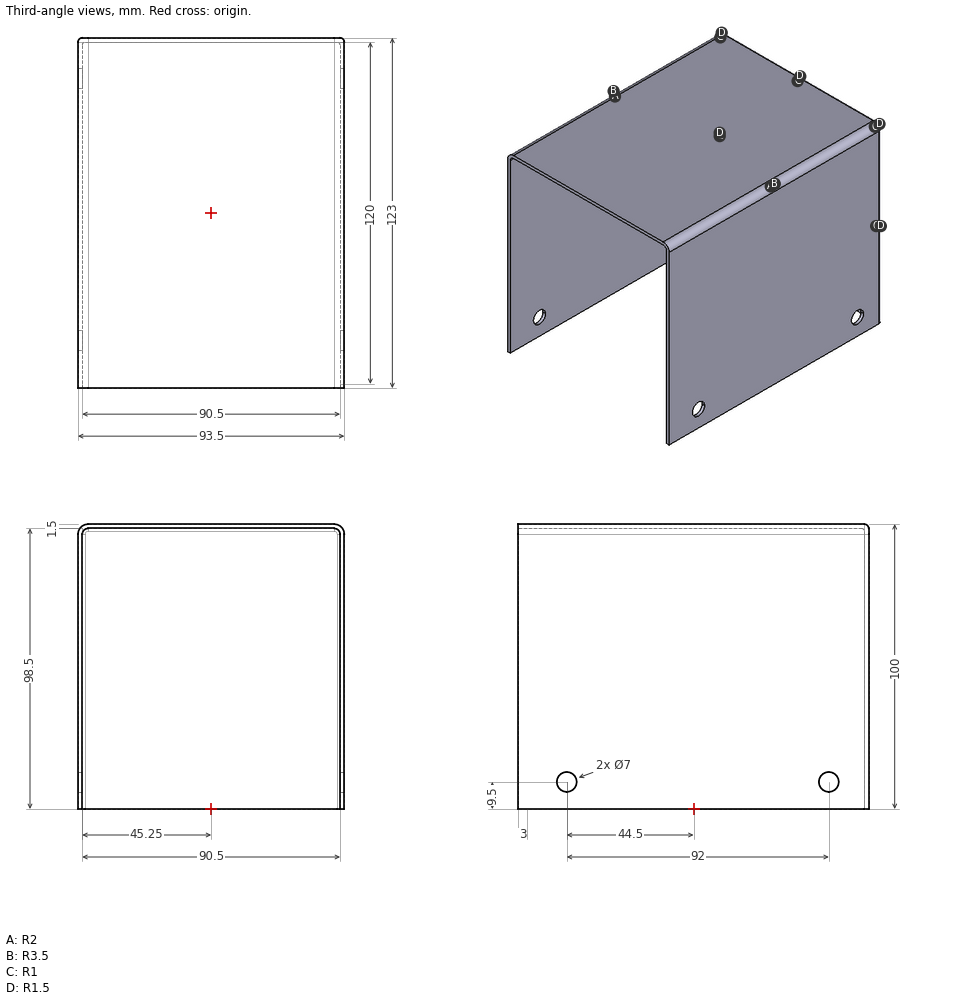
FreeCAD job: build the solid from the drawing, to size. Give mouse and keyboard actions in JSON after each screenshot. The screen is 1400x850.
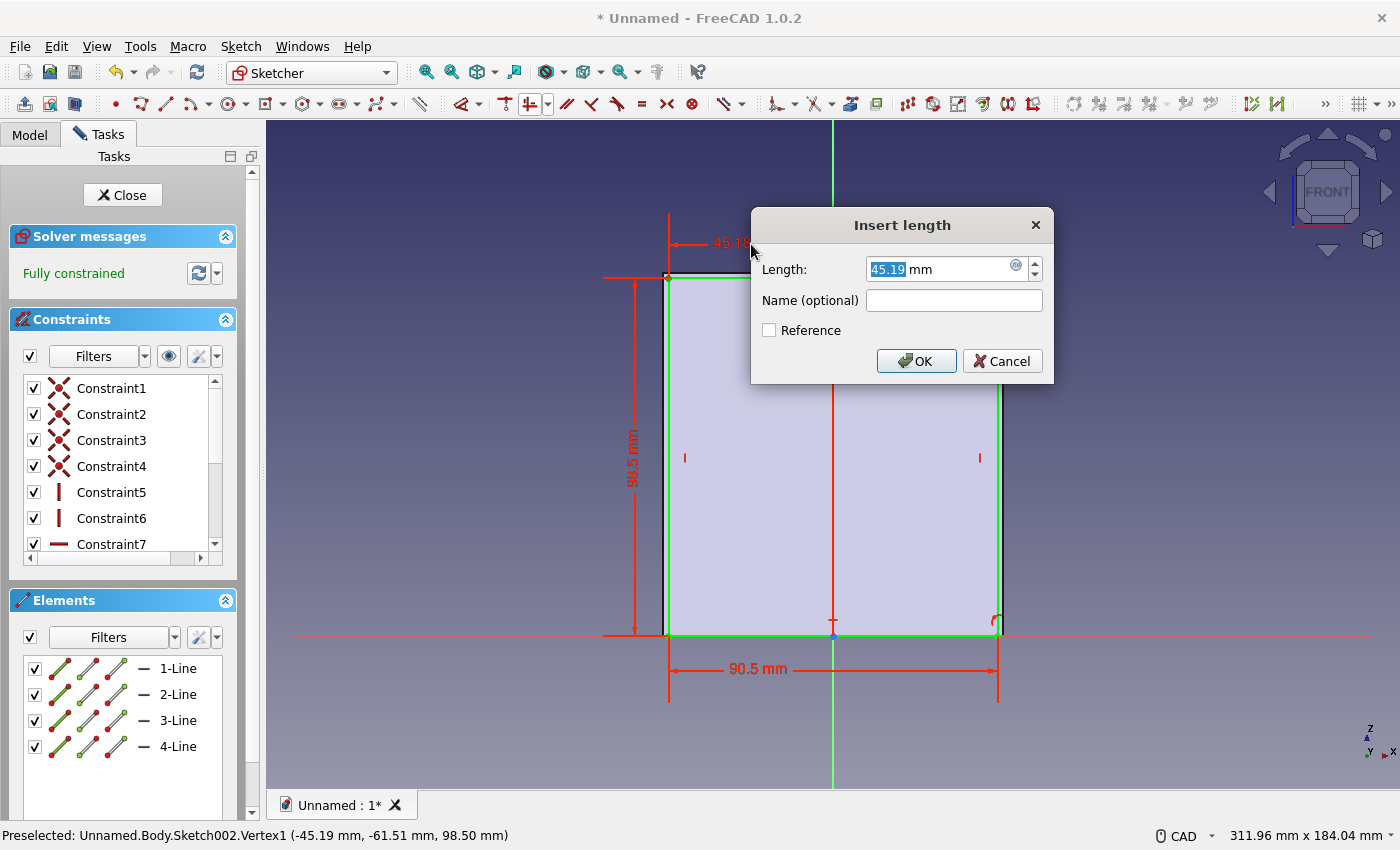
{"action": "type", "text": "45.25"}
{"action": "key", "text": "Return"}
{"action": "key", "text": "Escape"}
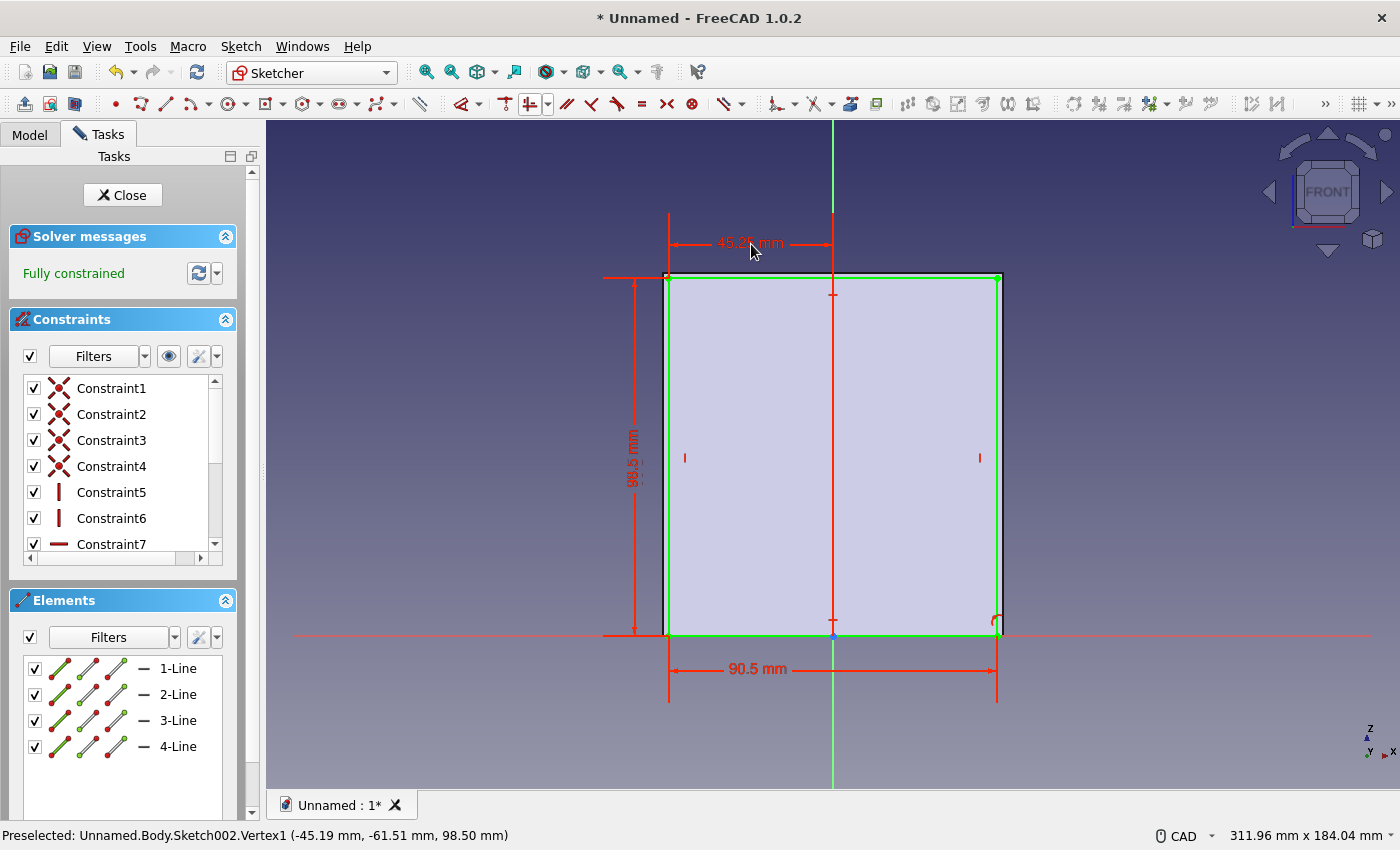
{"action": "left_click", "coordinate": [123, 195]}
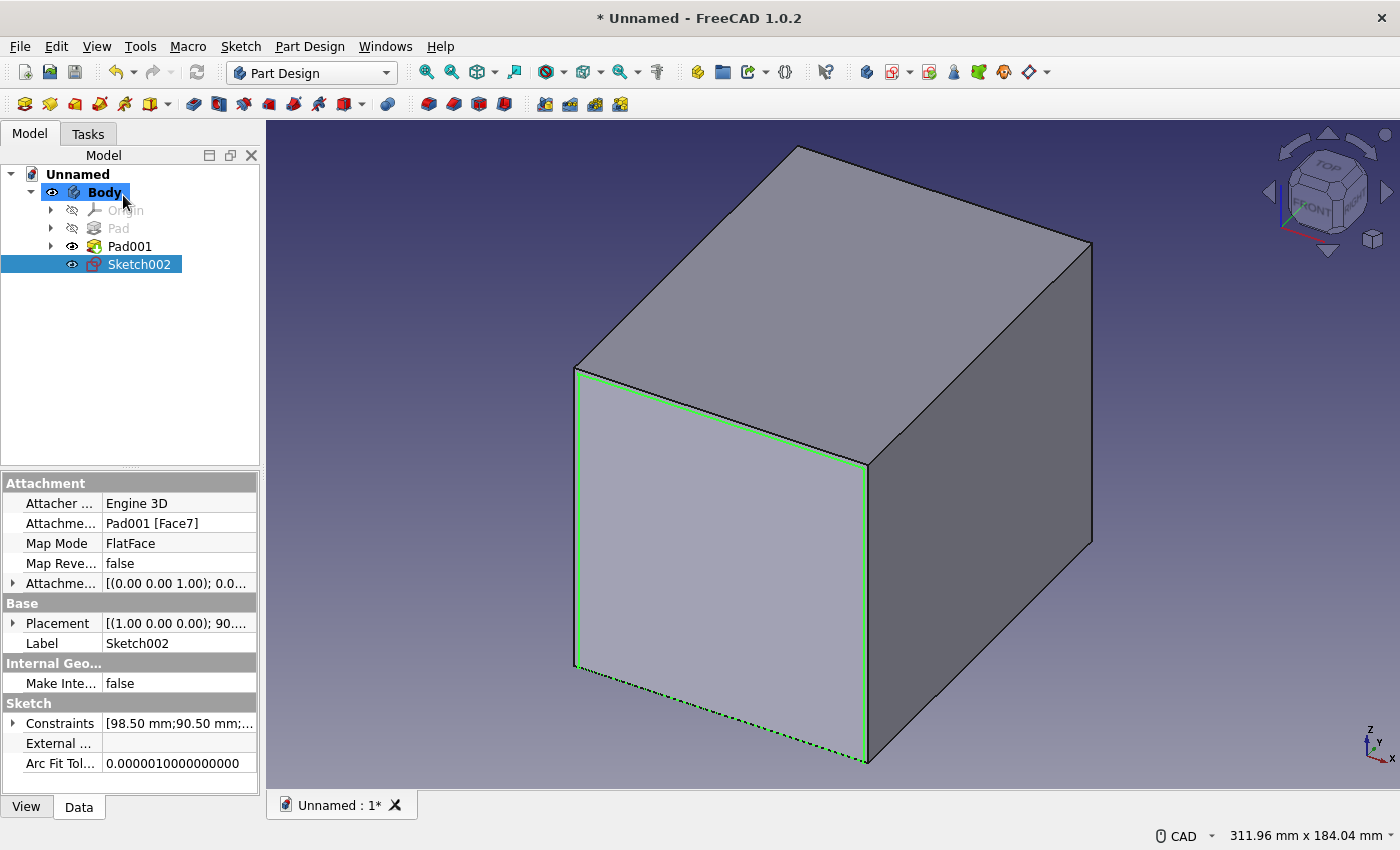
{"action": "left_click", "coordinate": [194, 104]}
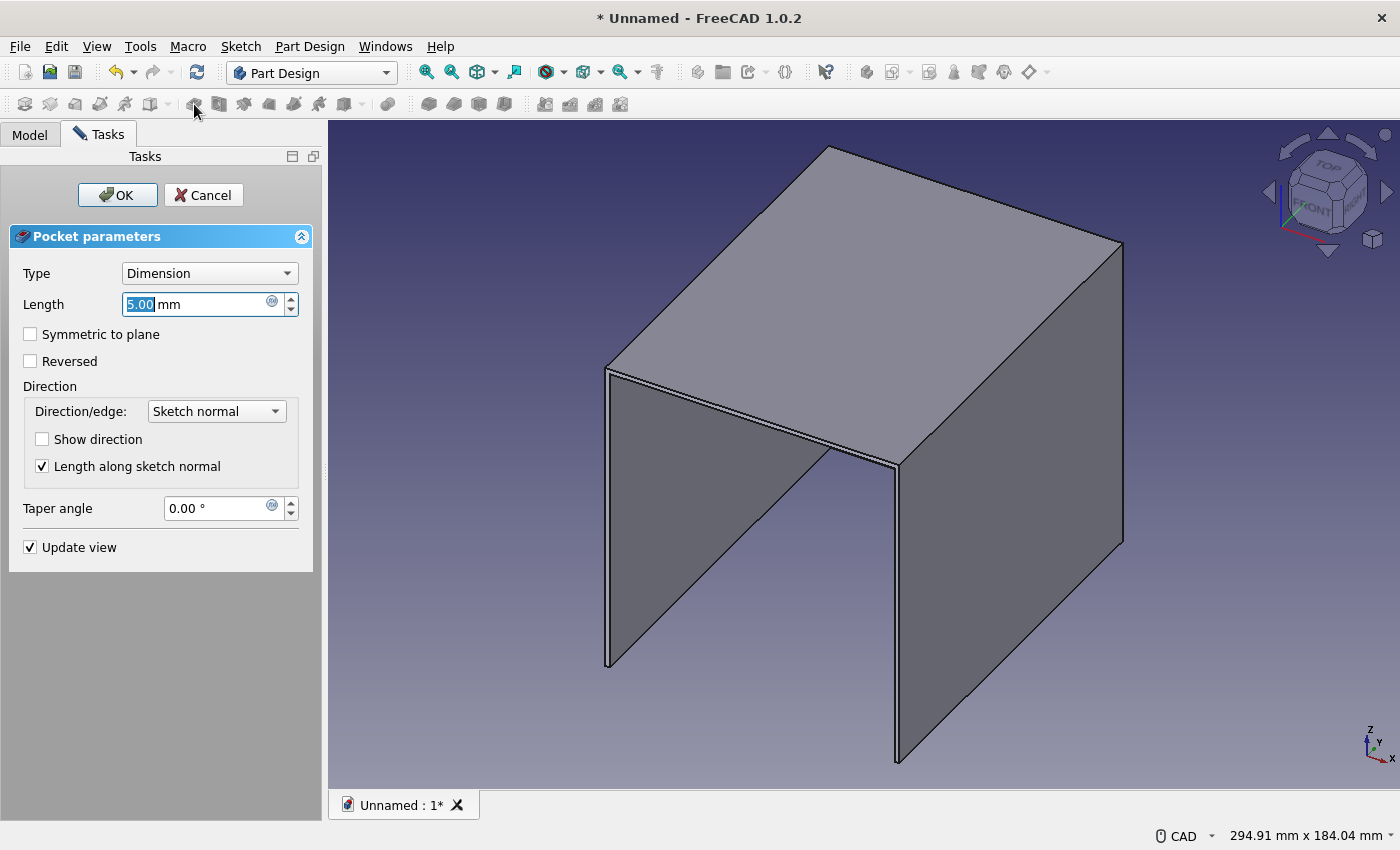
{"action": "type", "text": "3"}
{"action": "key", "text": "Tab"}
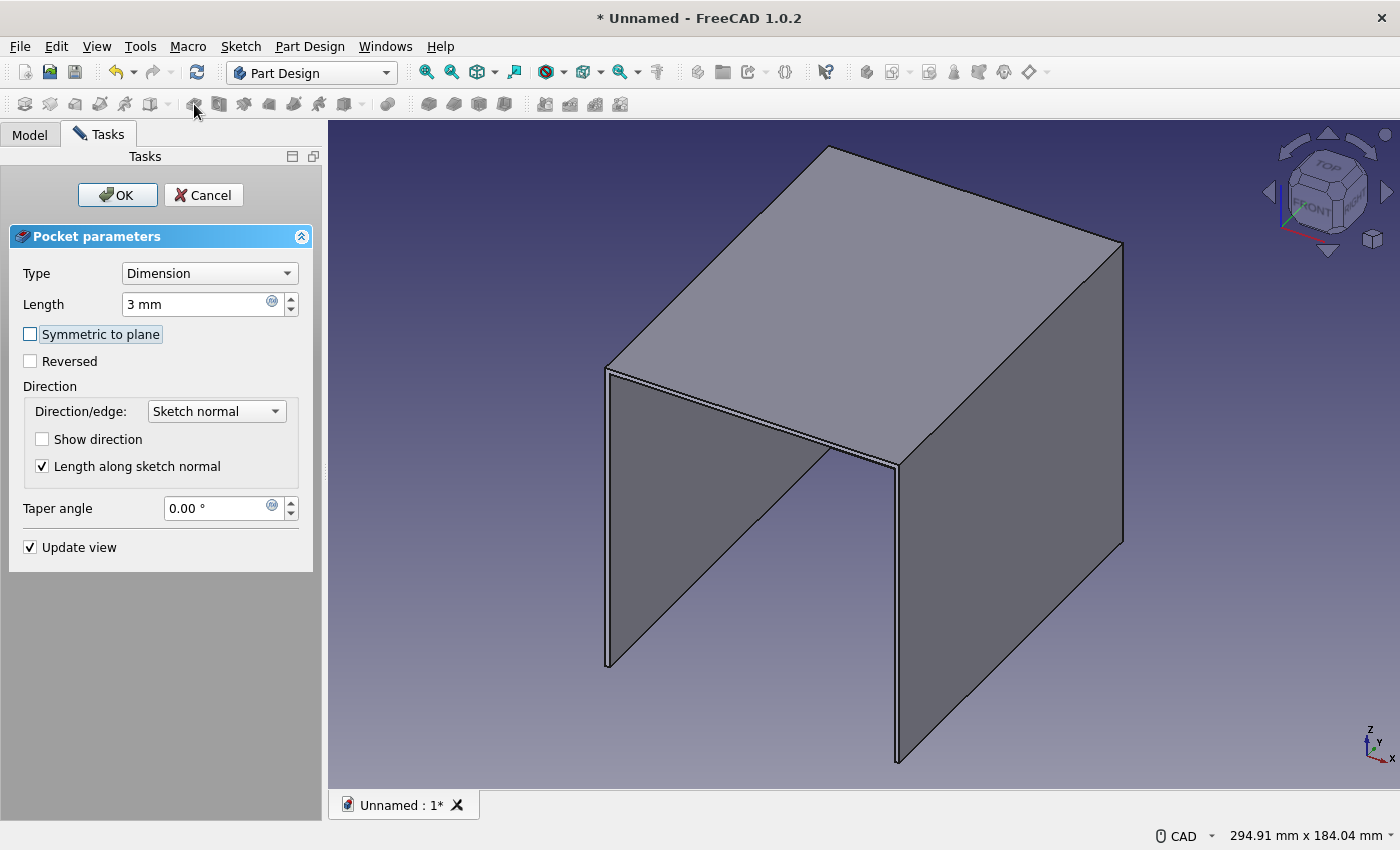
{"action": "left_click", "coordinate": [118, 195]}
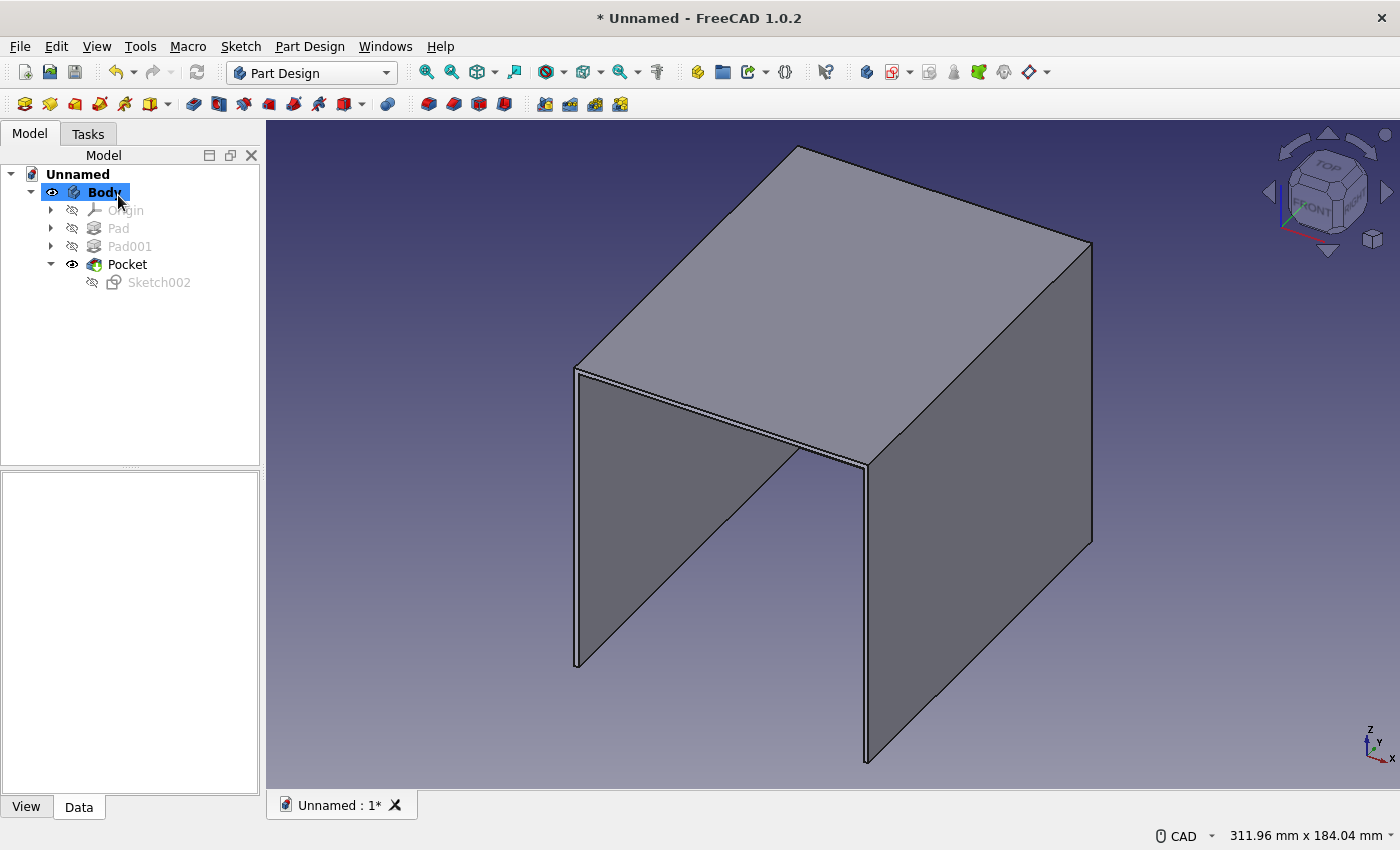
{"action": "left_click", "coordinate": [980, 502]}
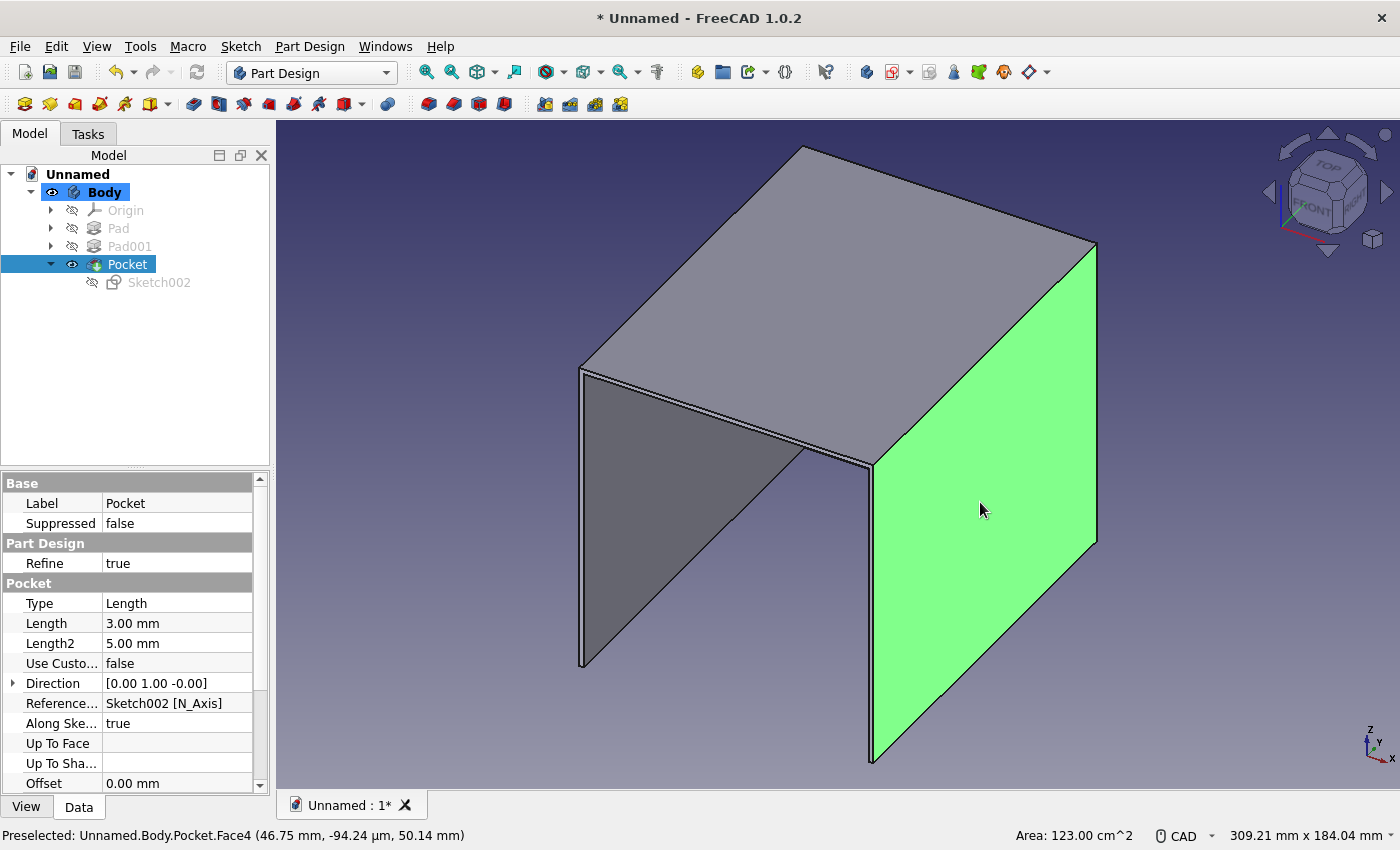
{"action": "left_click", "coordinate": [892, 72]}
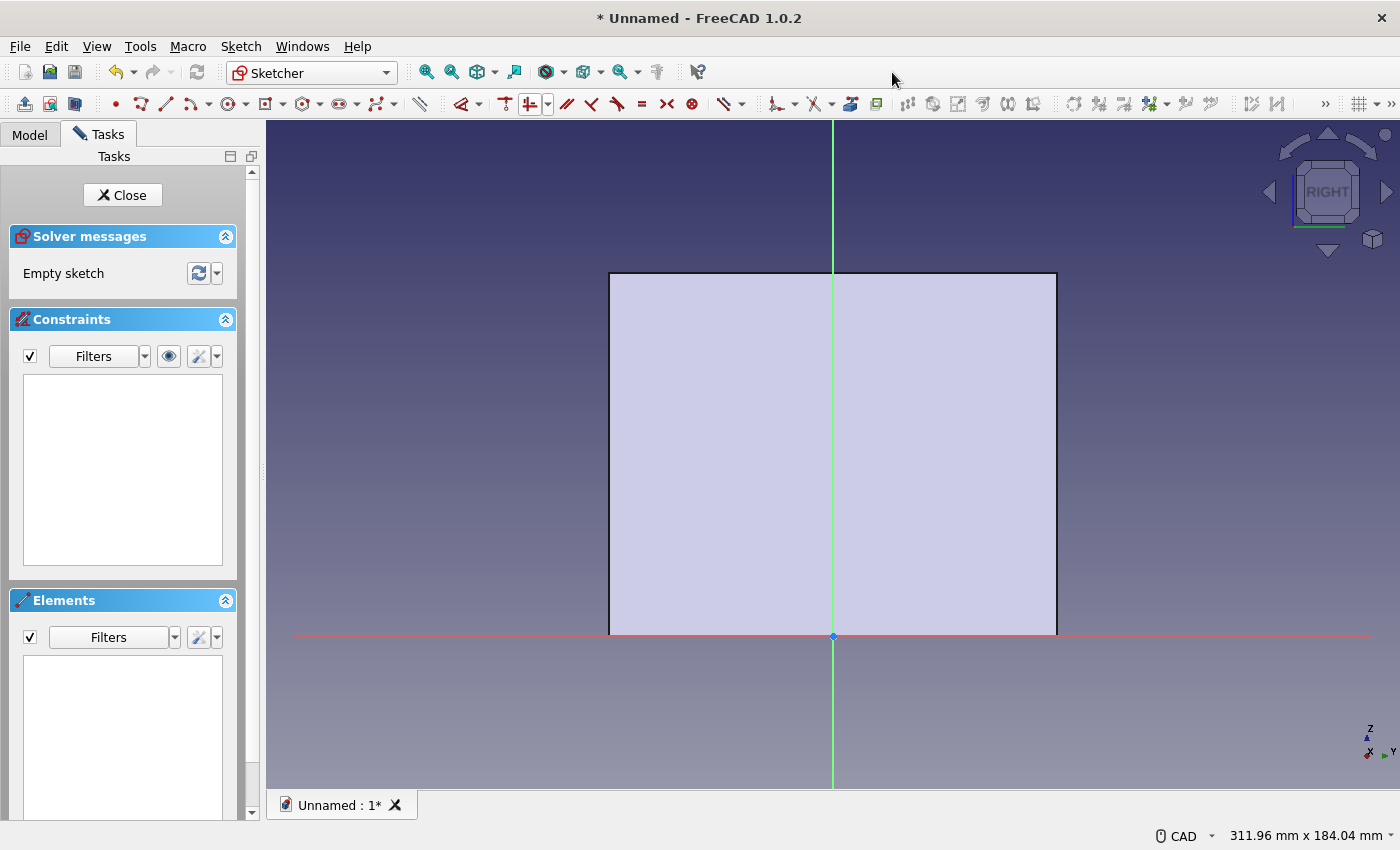
{"action": "scroll", "coordinate": [928, 761], "scroll_direction": "up", "scroll_amount": 3}